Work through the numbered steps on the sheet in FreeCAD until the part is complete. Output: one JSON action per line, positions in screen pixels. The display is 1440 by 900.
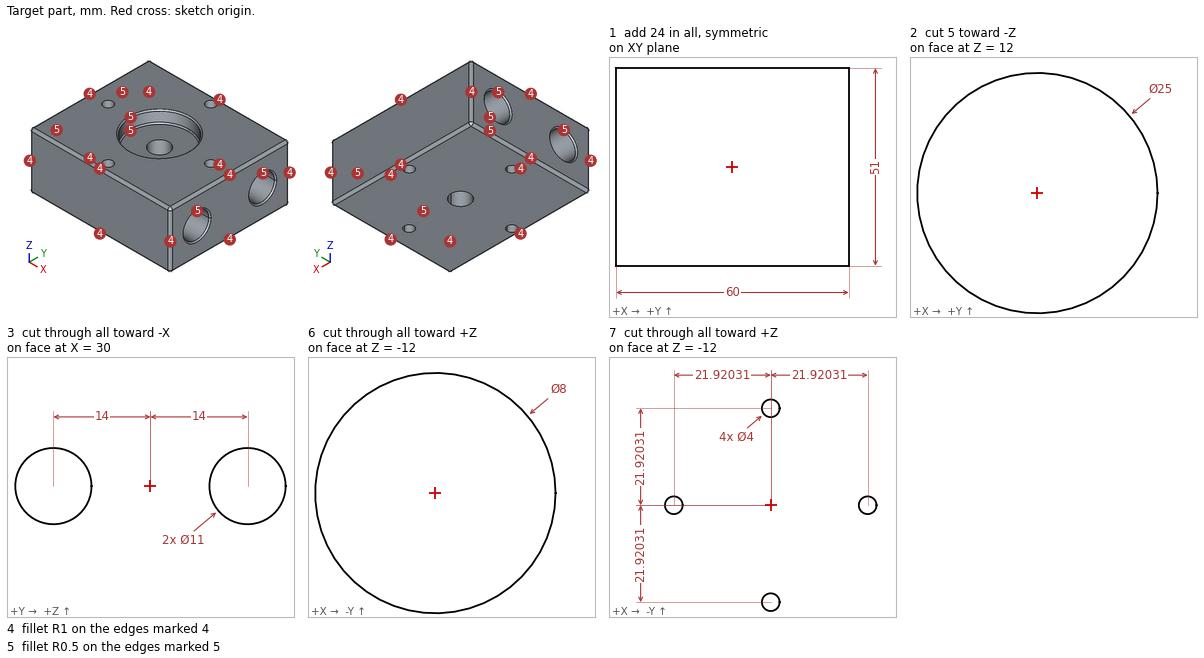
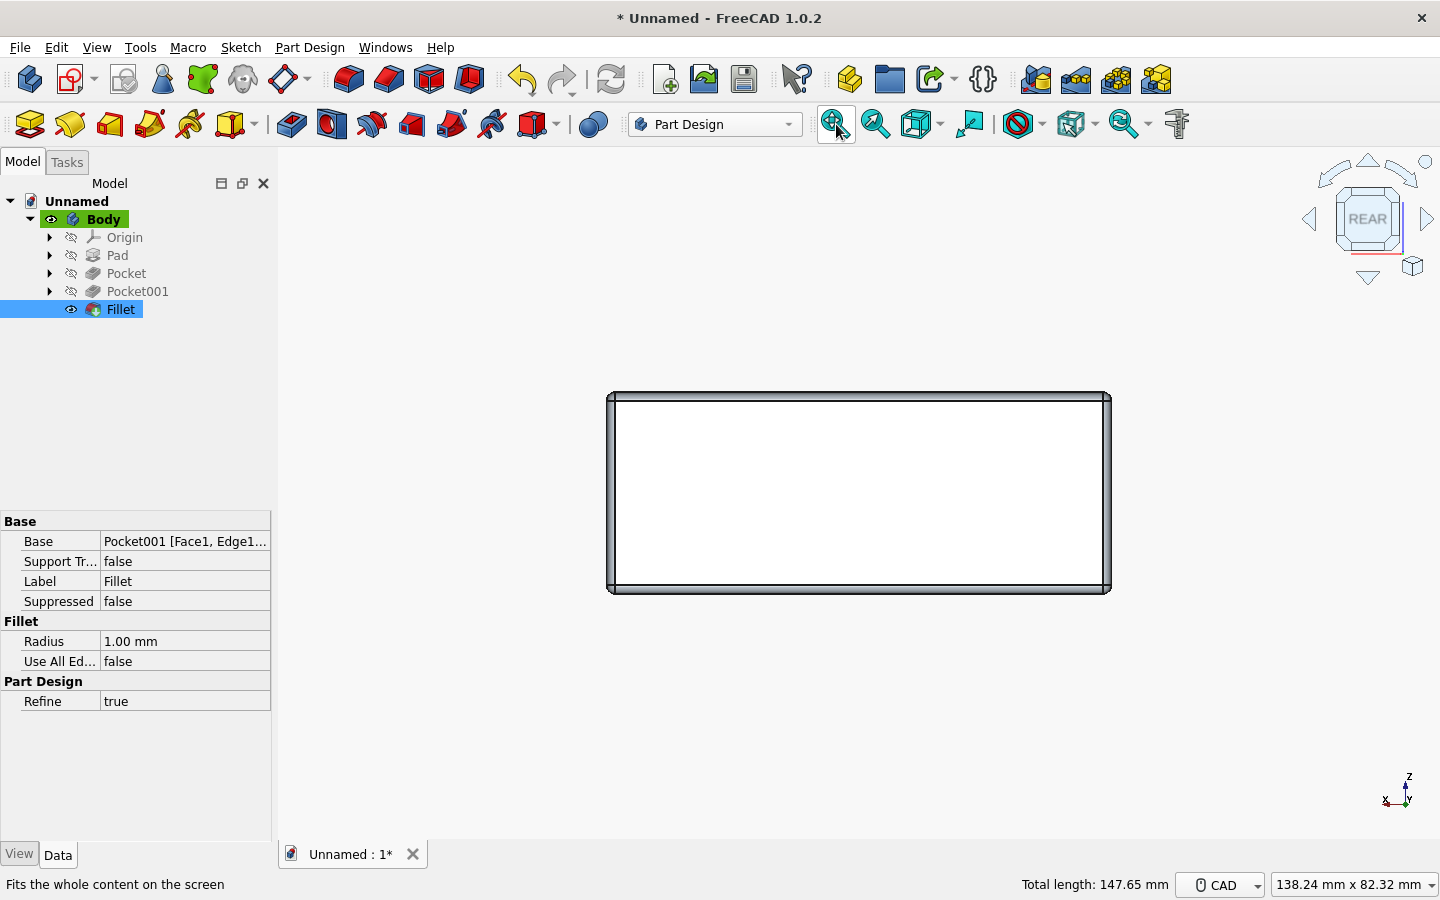
{"action": "key", "text": "6"}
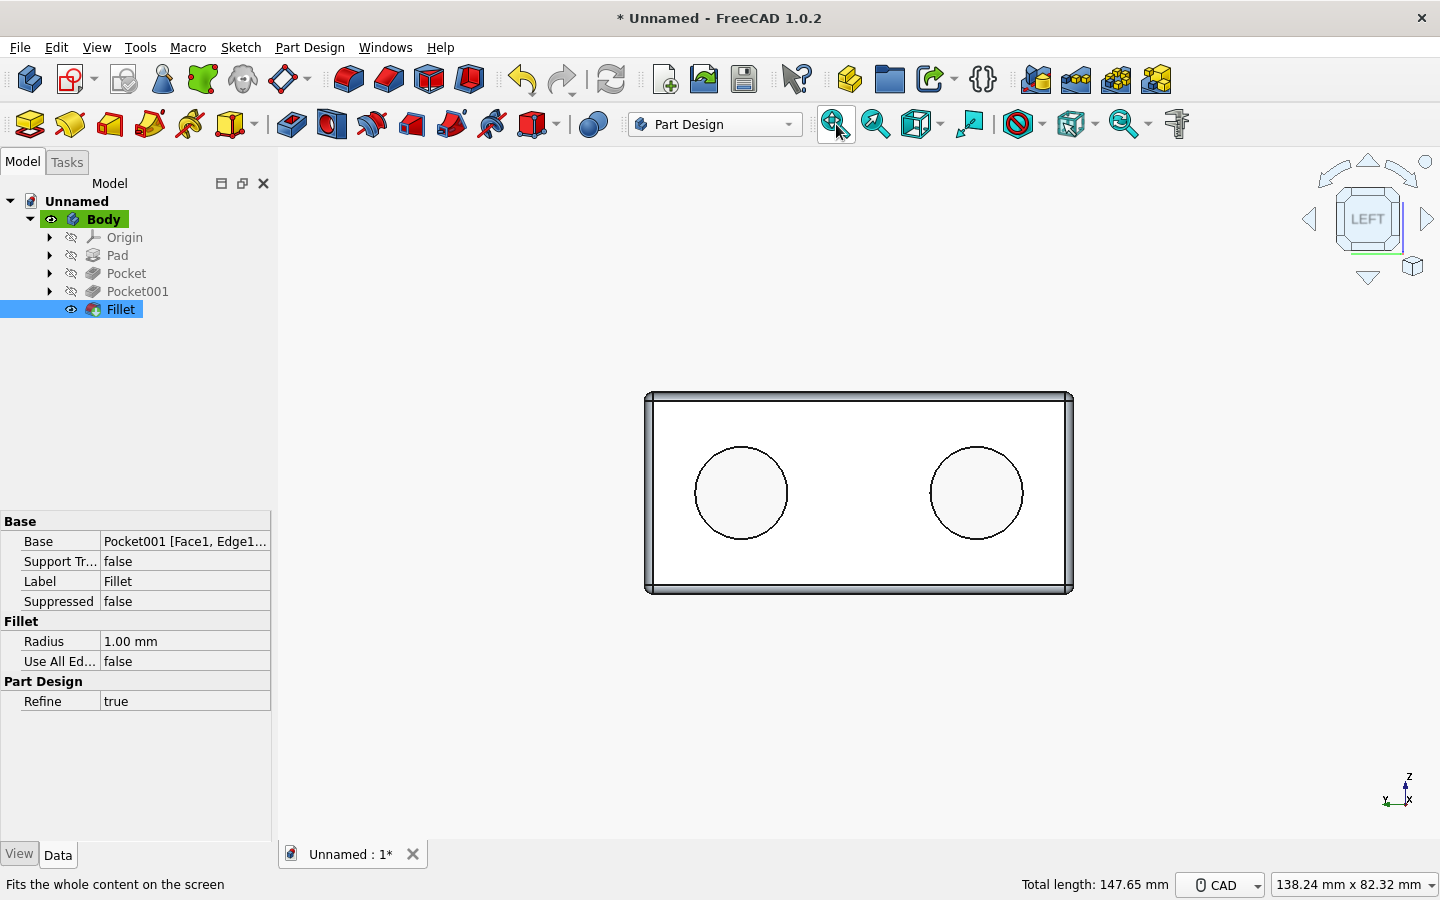
{"action": "left_click", "coordinate": [836, 124]}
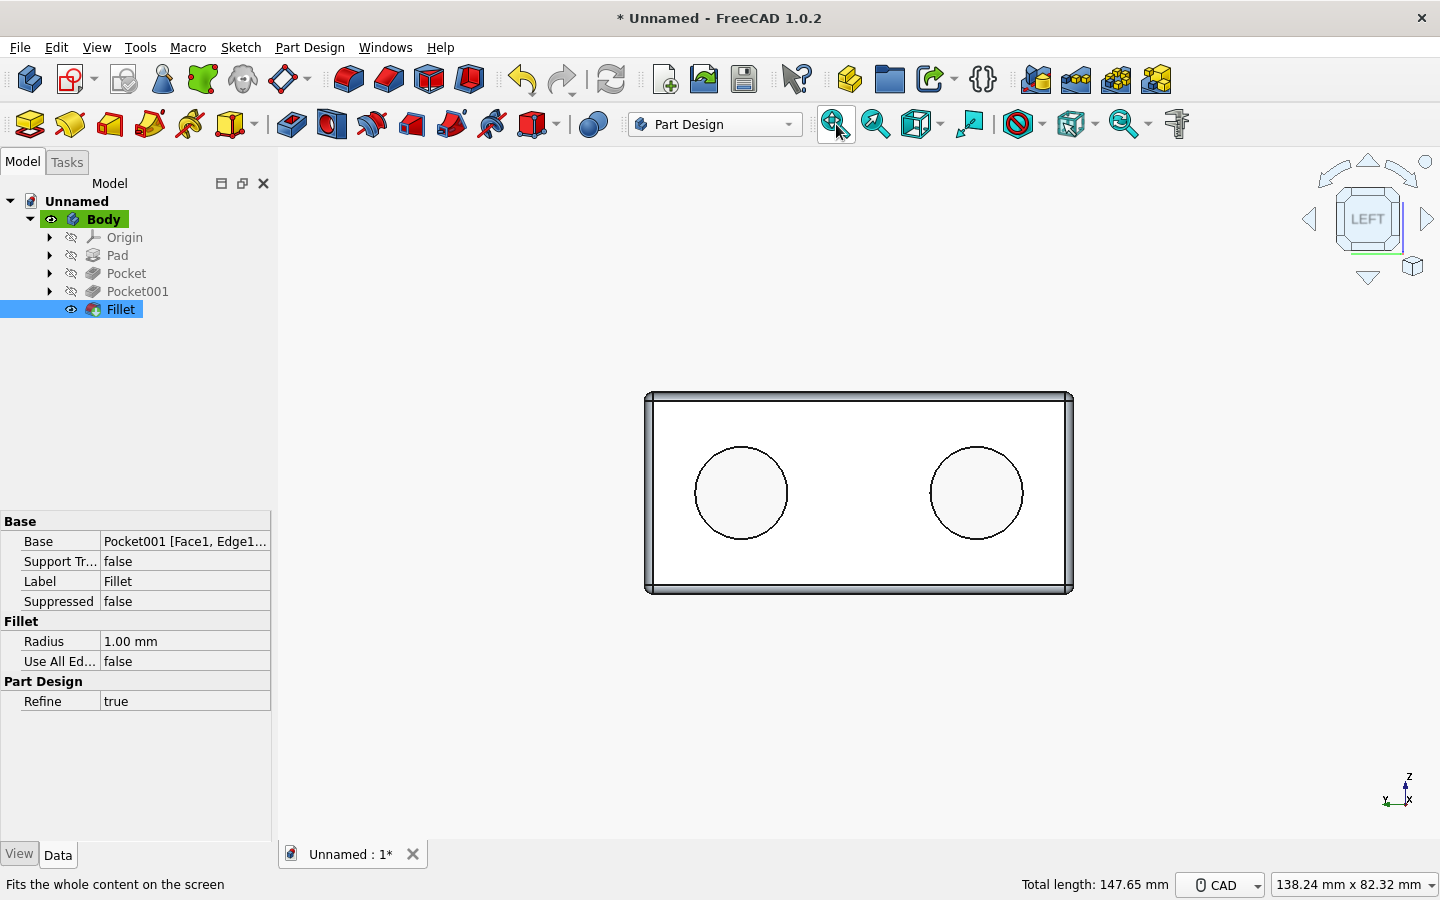
{"action": "left_click", "coordinate": [788, 492], "text": "ctrl"}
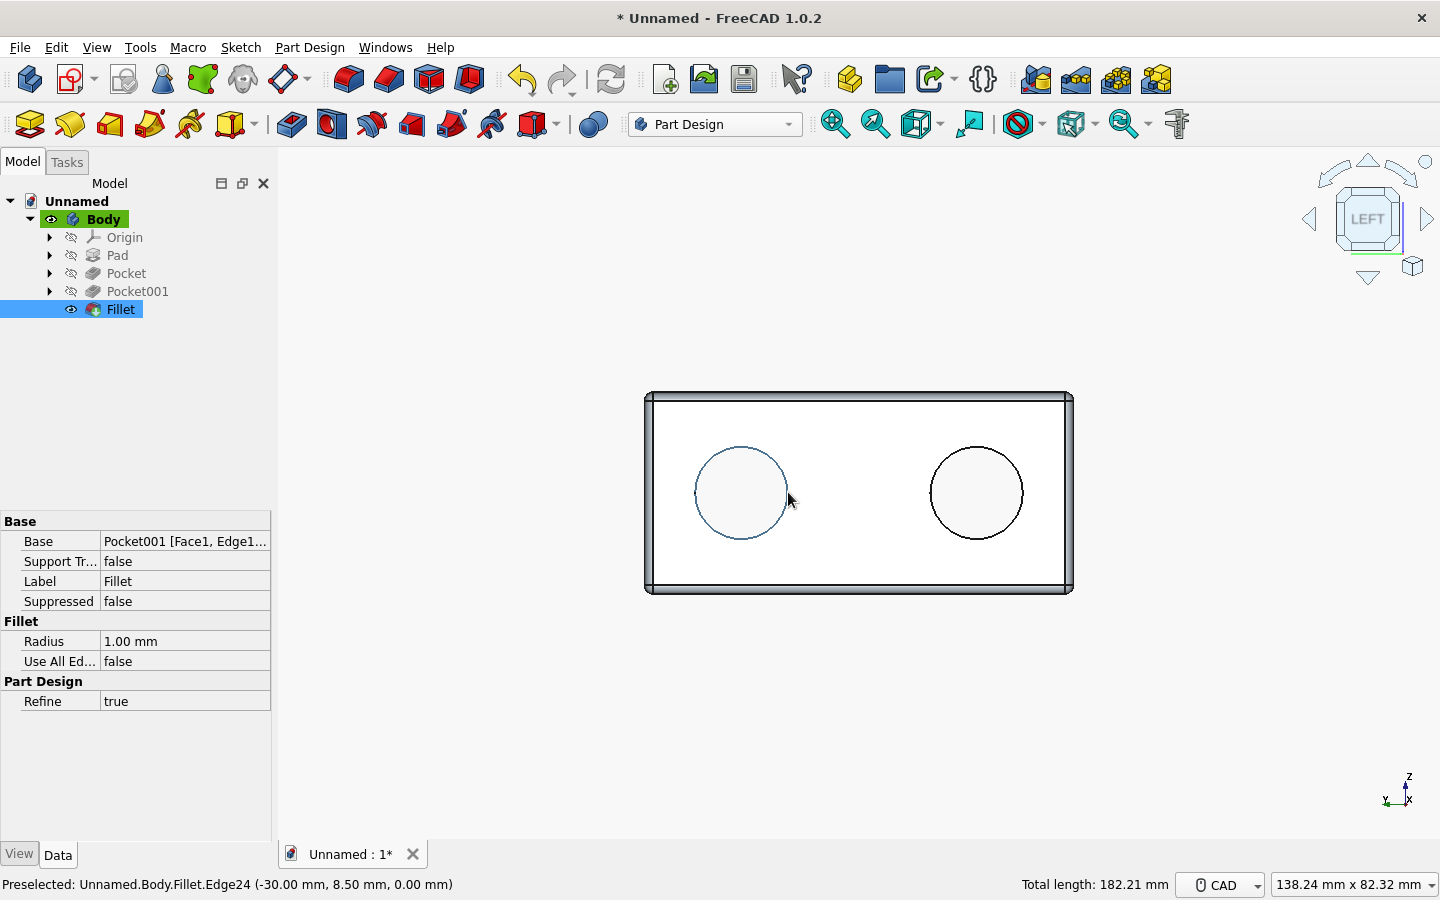
{"action": "left_click", "coordinate": [1023, 492], "text": "ctrl"}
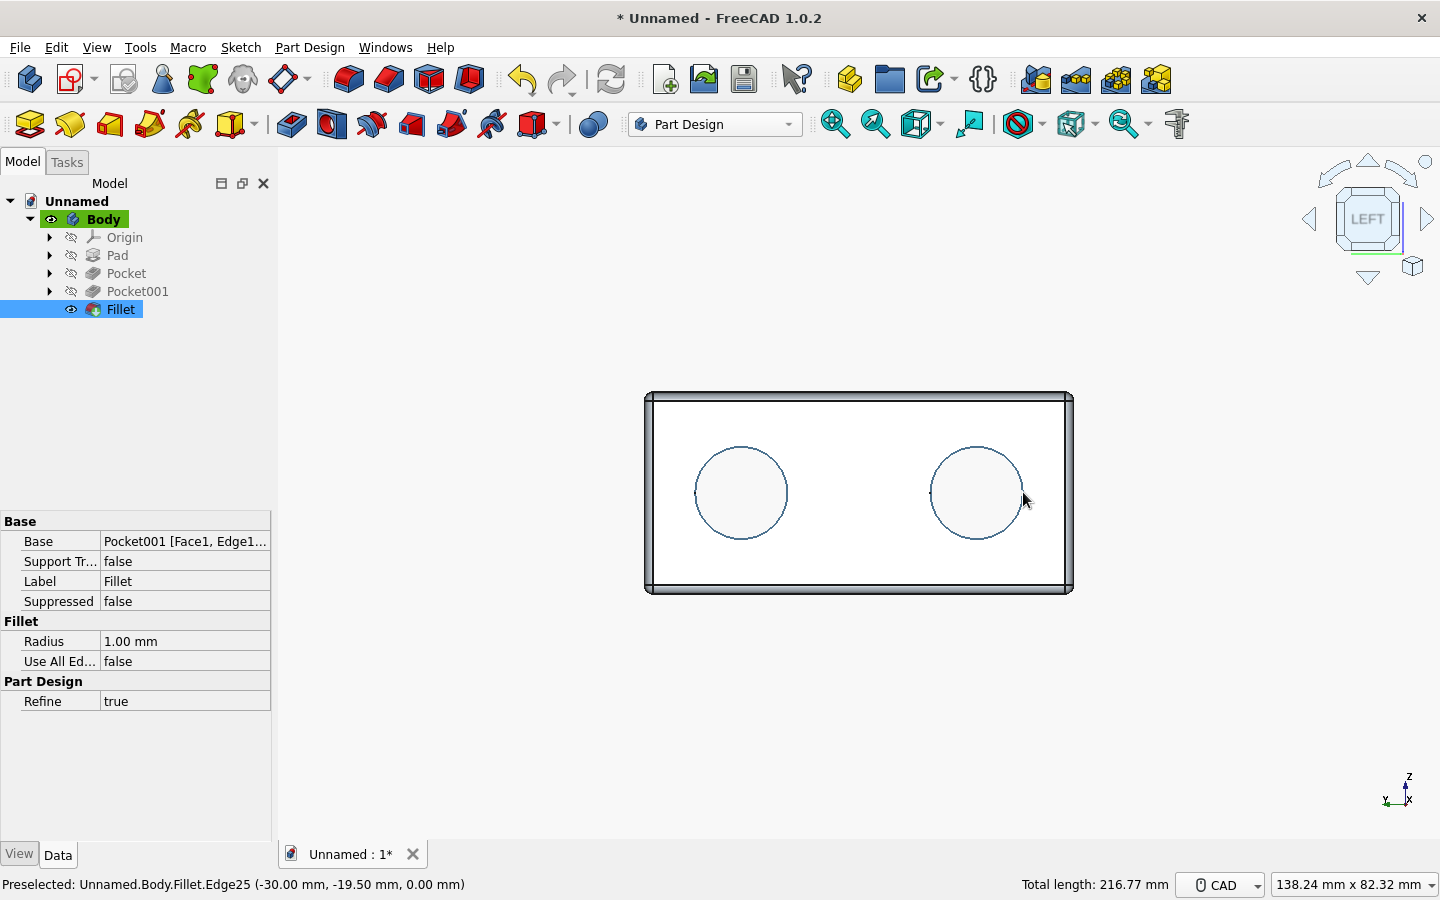
{"action": "key", "text": "v 3"}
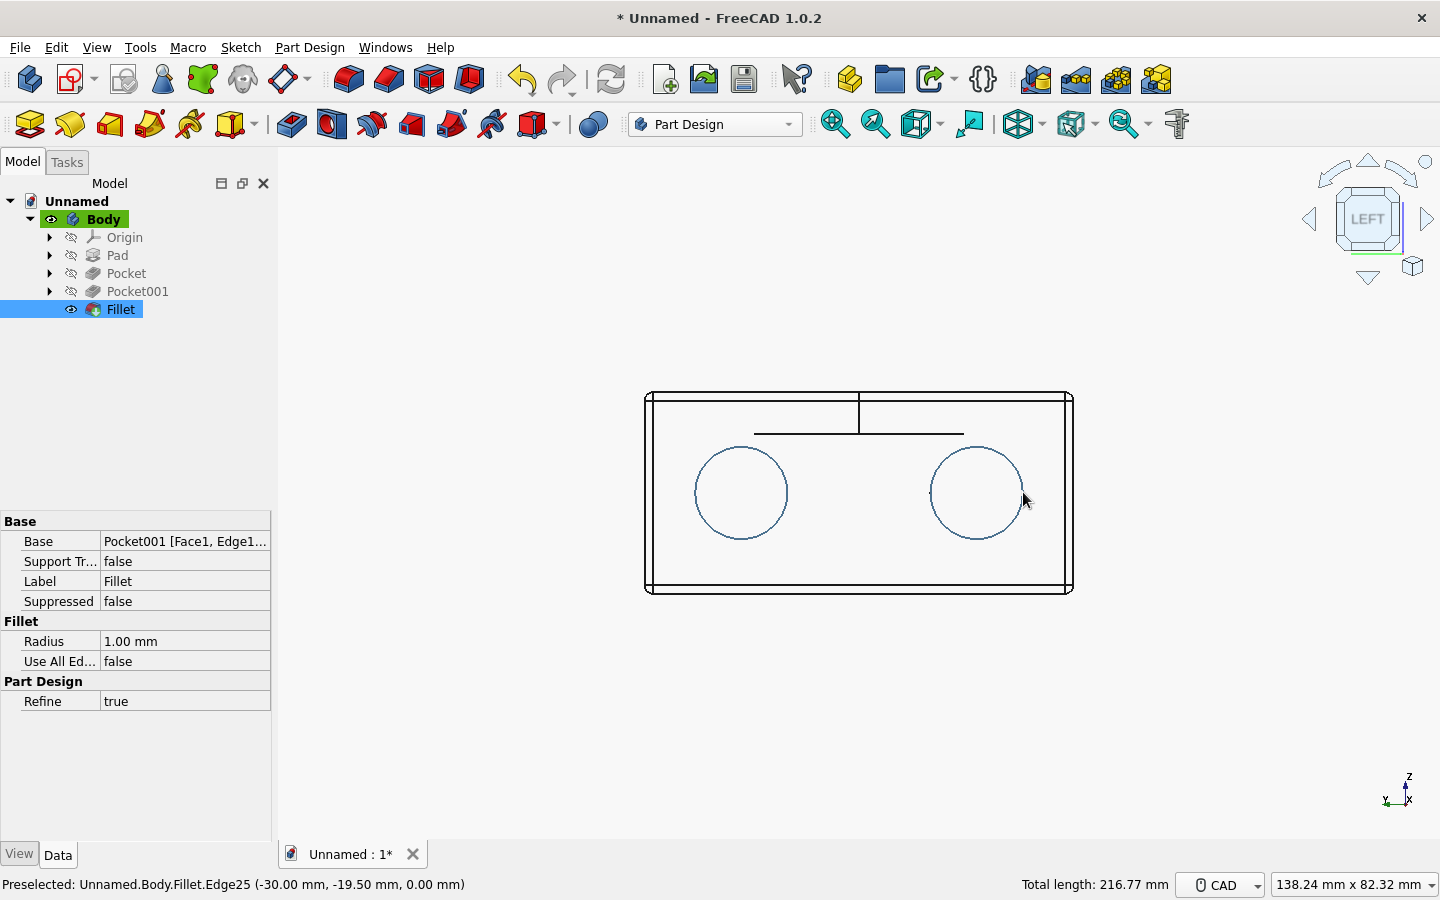
{"action": "key", "text": "0"}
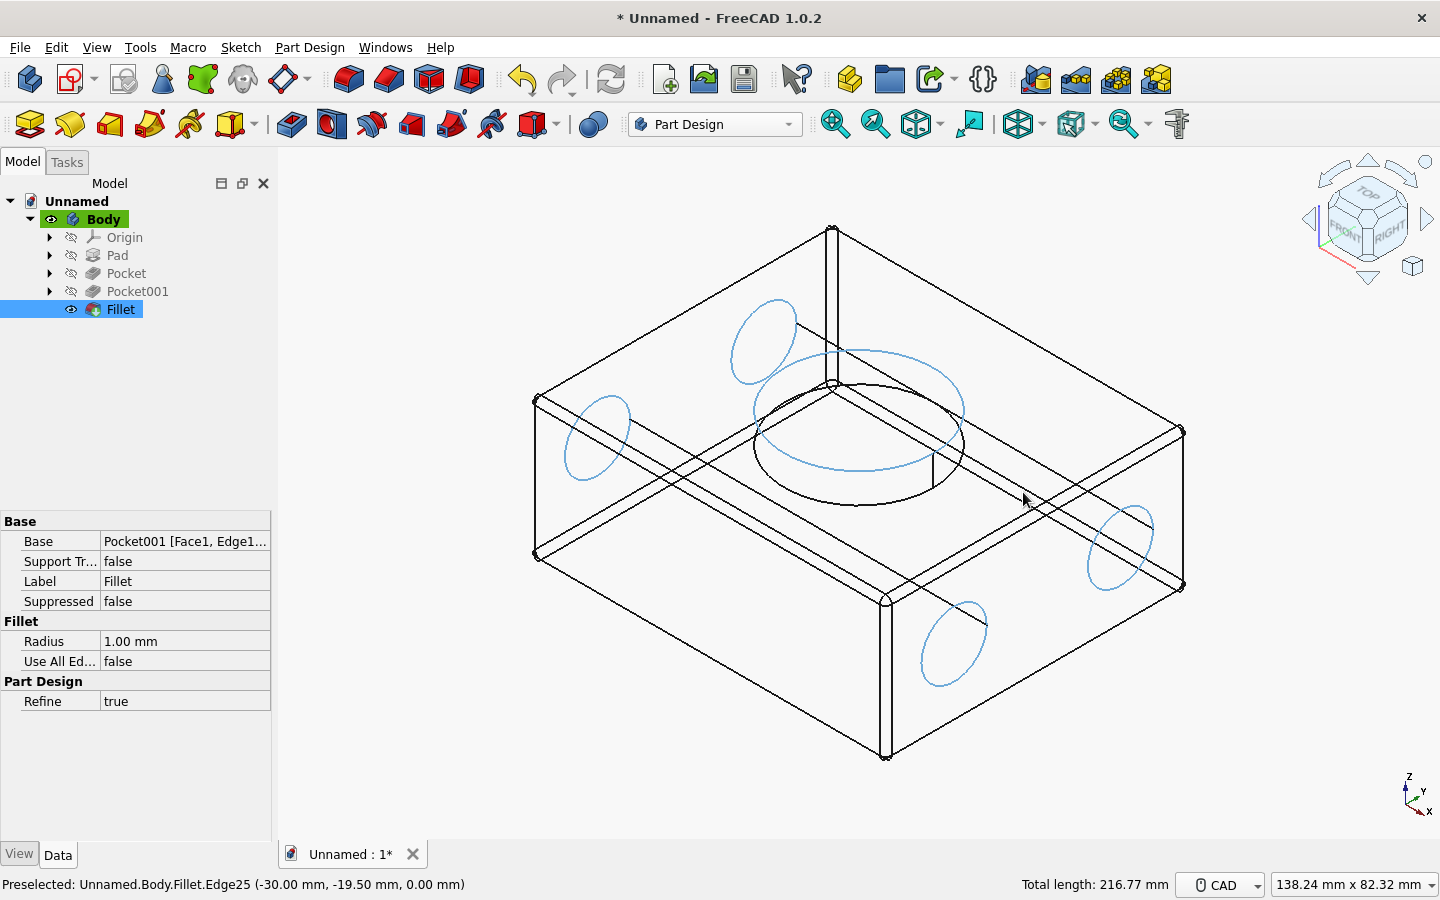
{"action": "left_click", "coordinate": [785, 401], "text": "ctrl"}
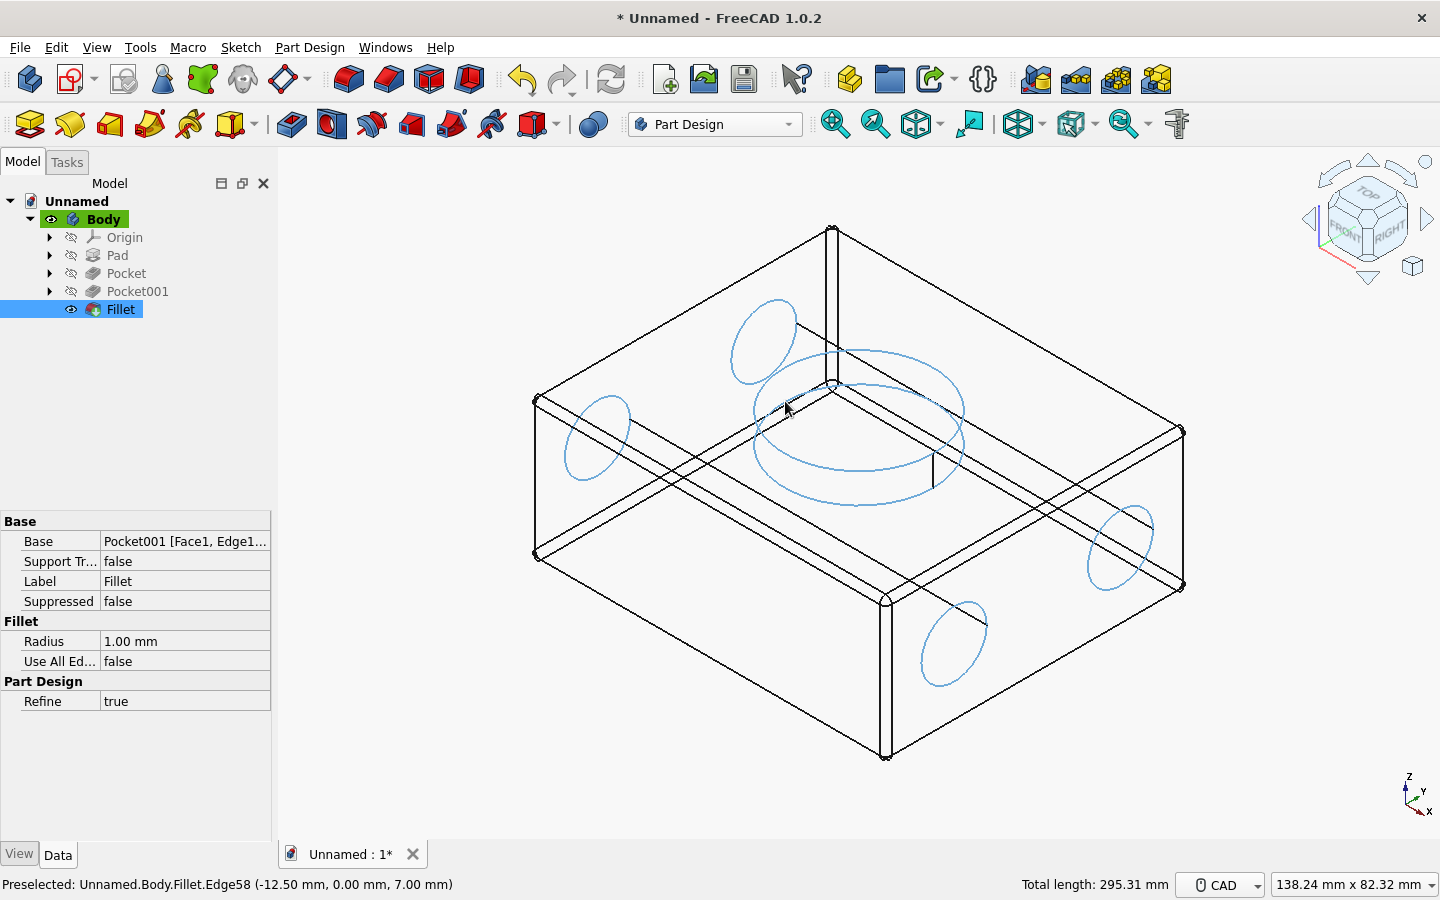
{"action": "key", "text": "v 1"}